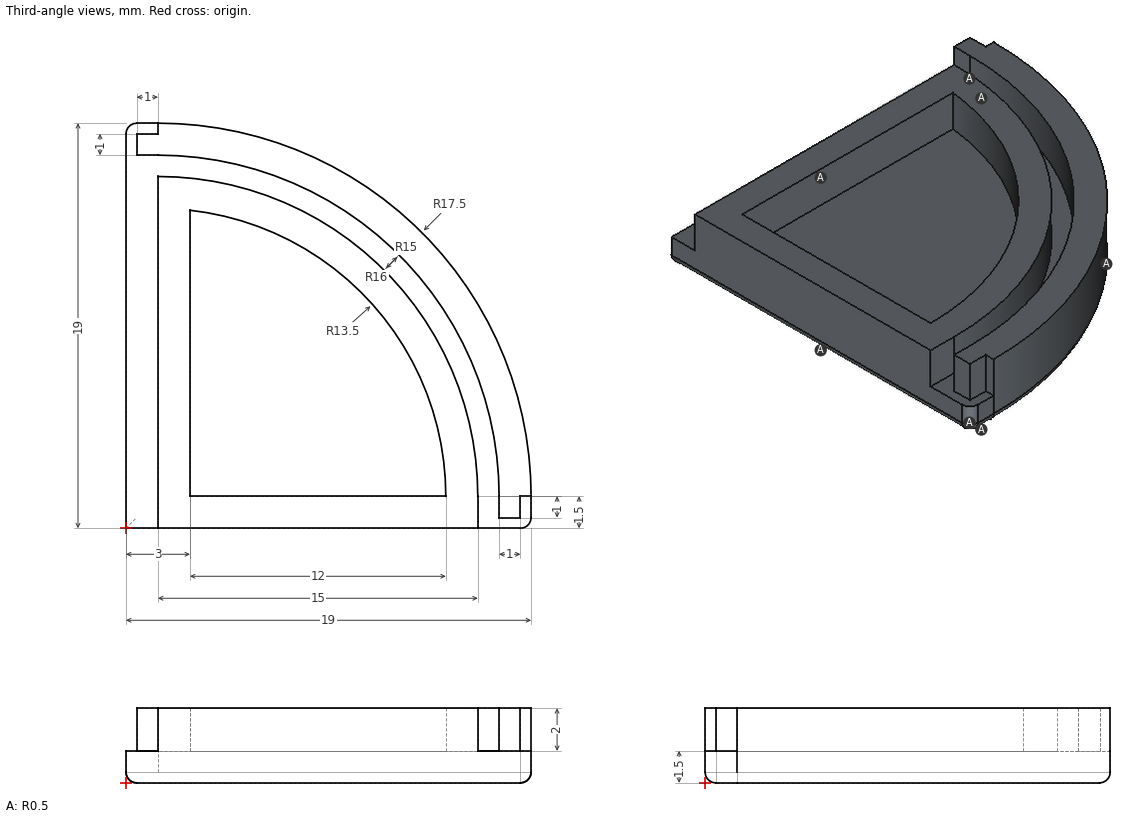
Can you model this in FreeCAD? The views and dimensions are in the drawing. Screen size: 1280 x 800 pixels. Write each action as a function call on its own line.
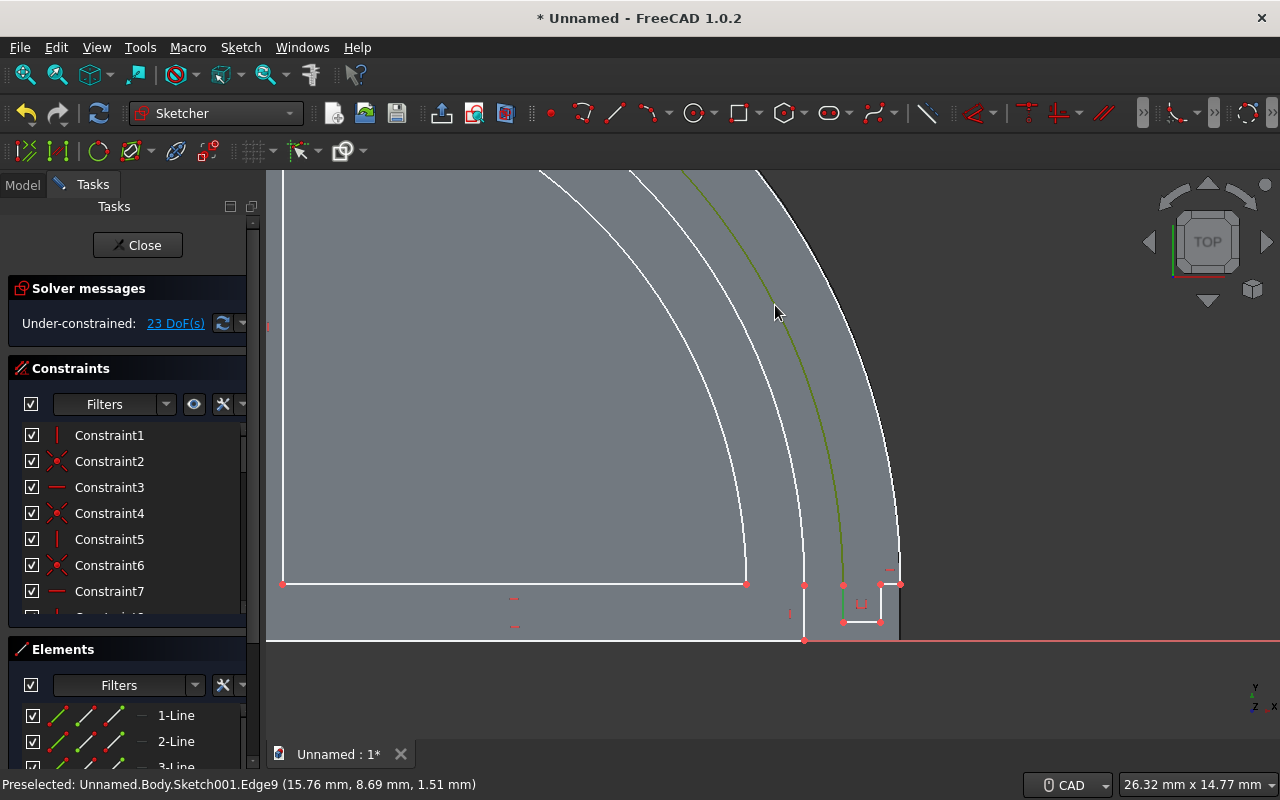
key(t)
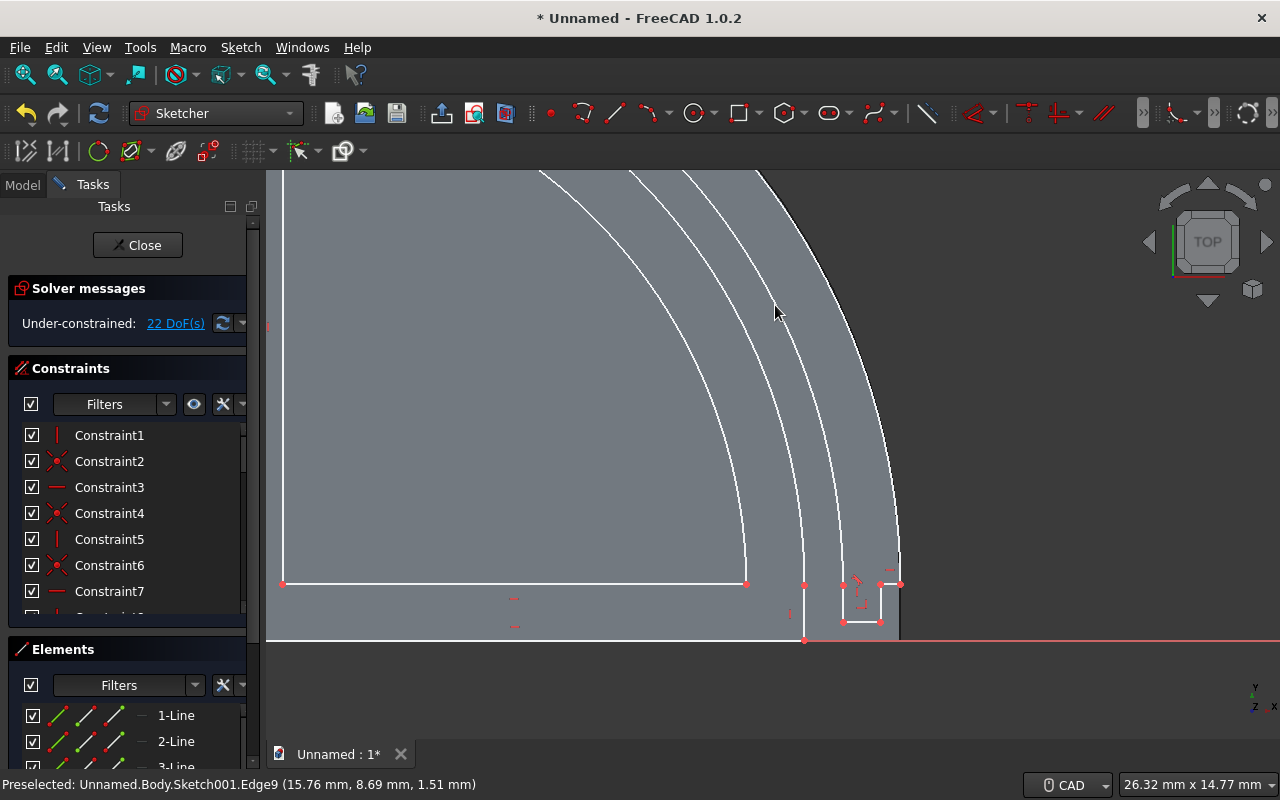
click(804, 624)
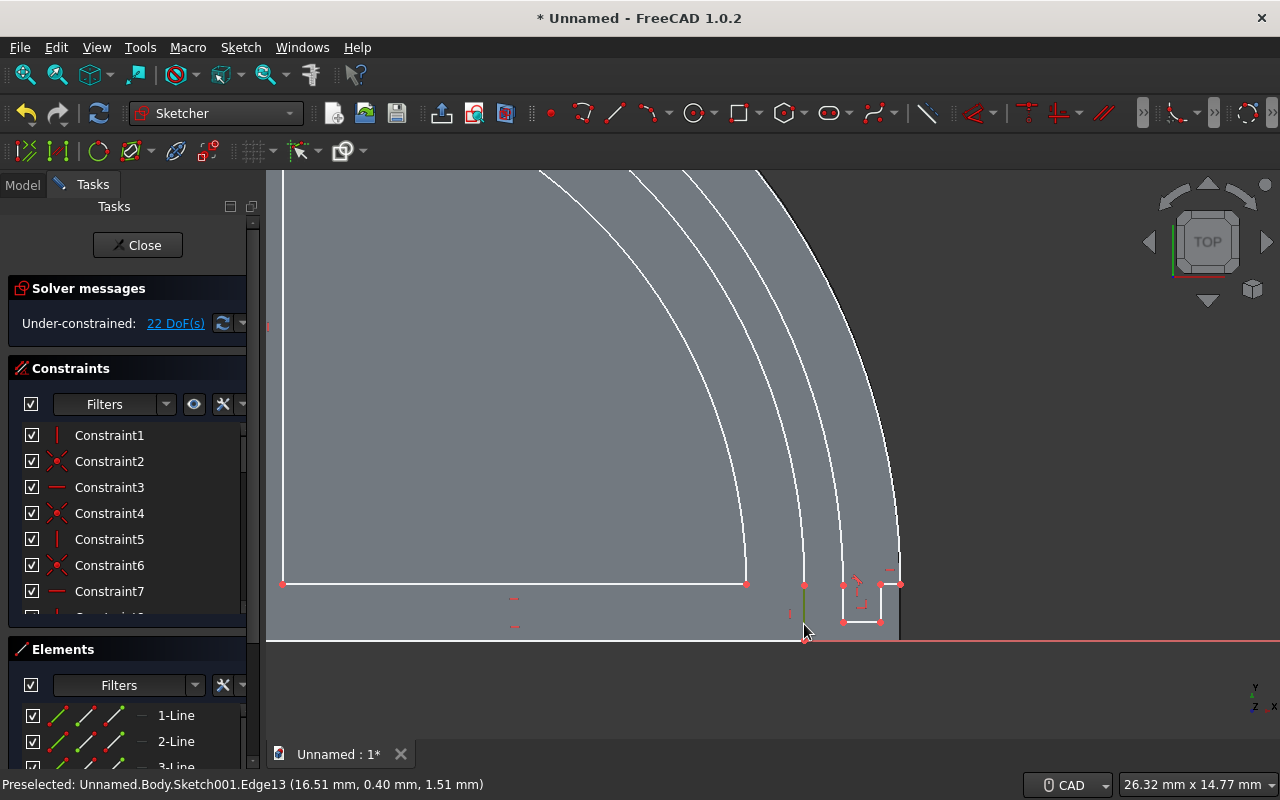
click(742, 323)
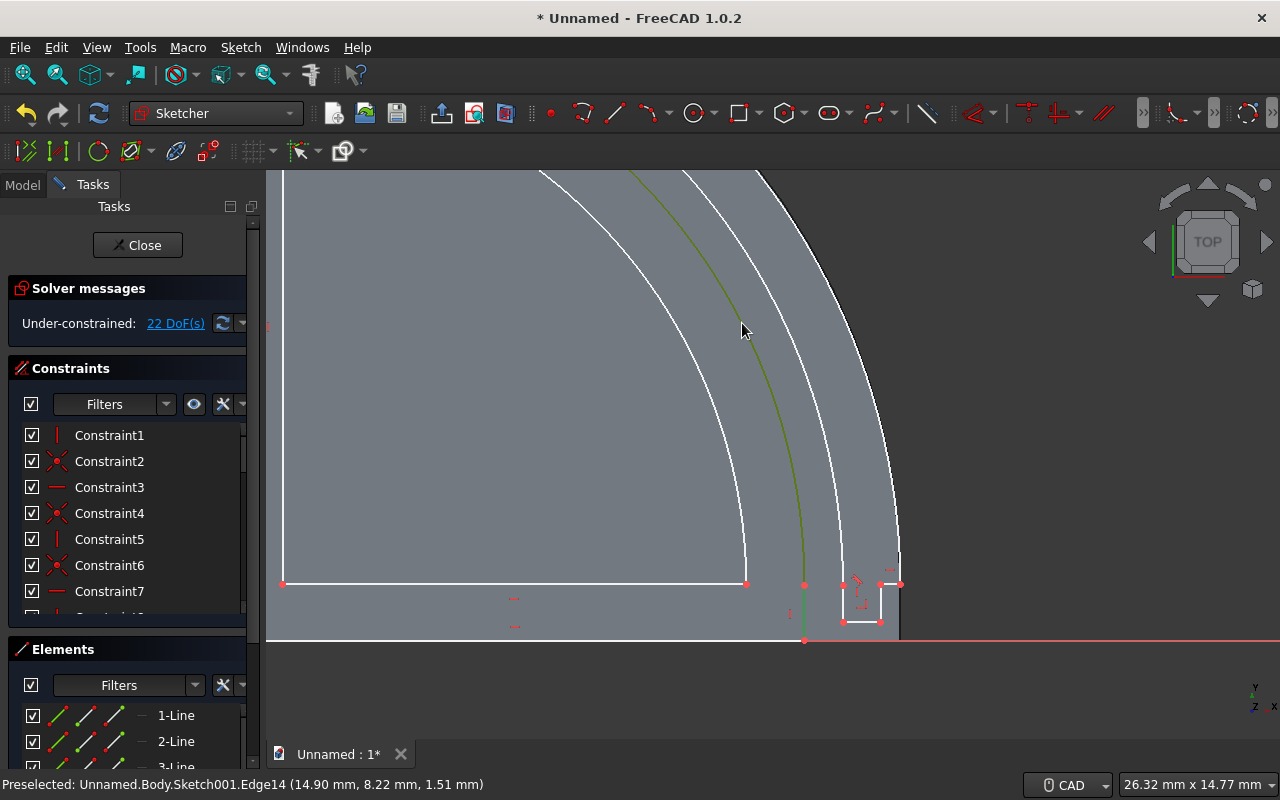
key(t)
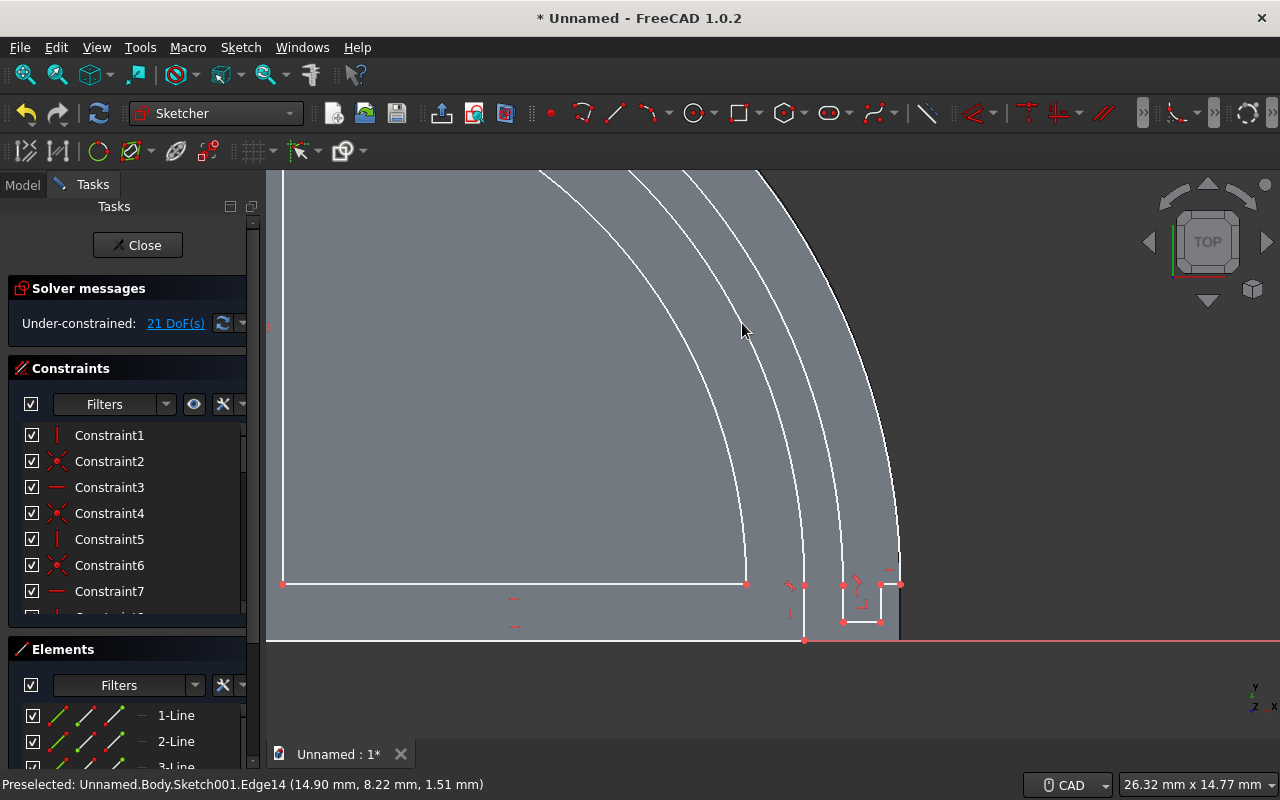
click(775, 304)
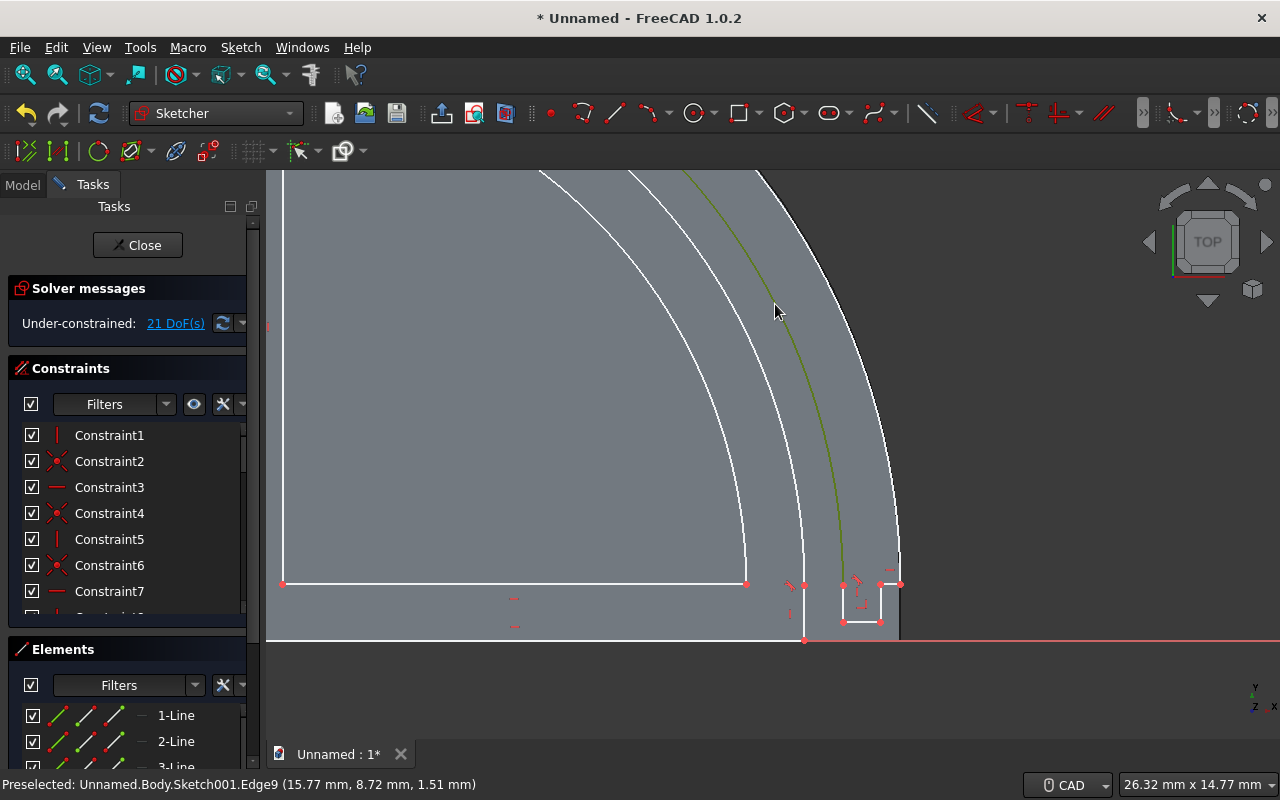
click(826, 279)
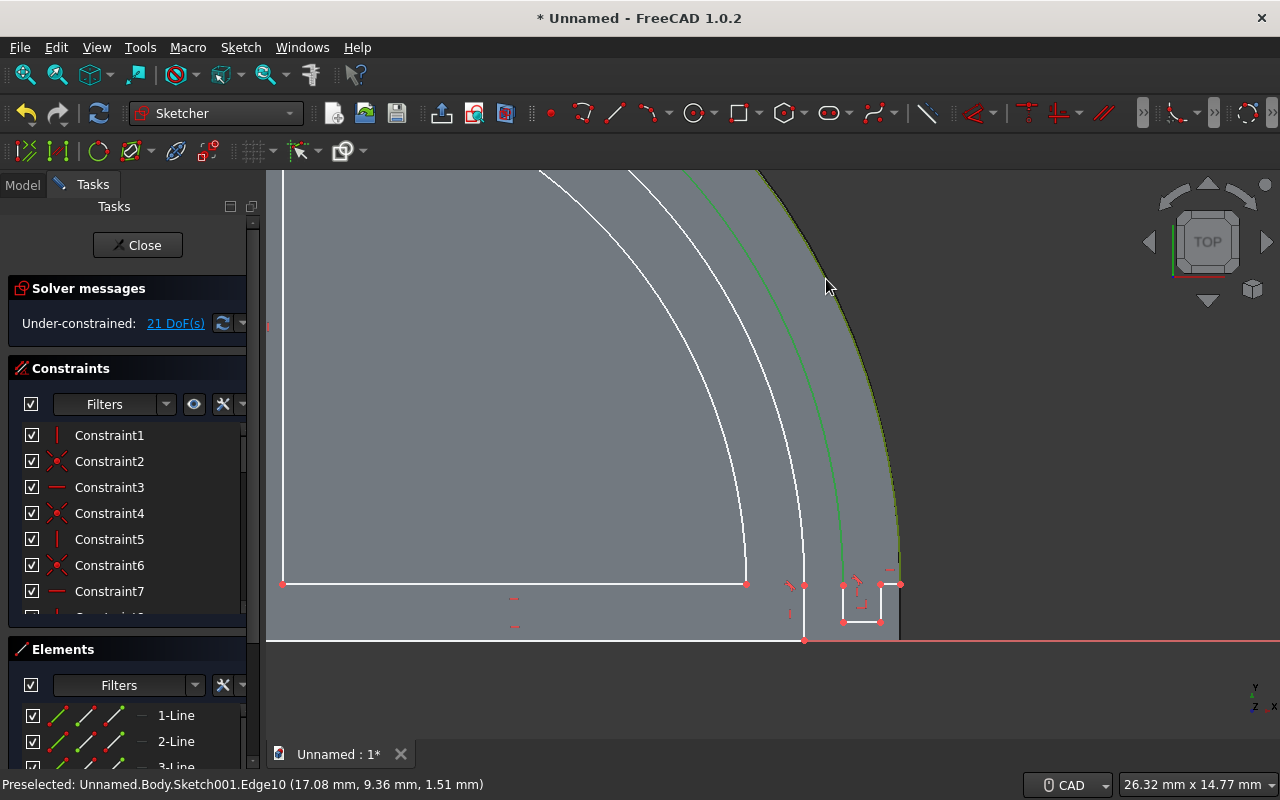
key(c)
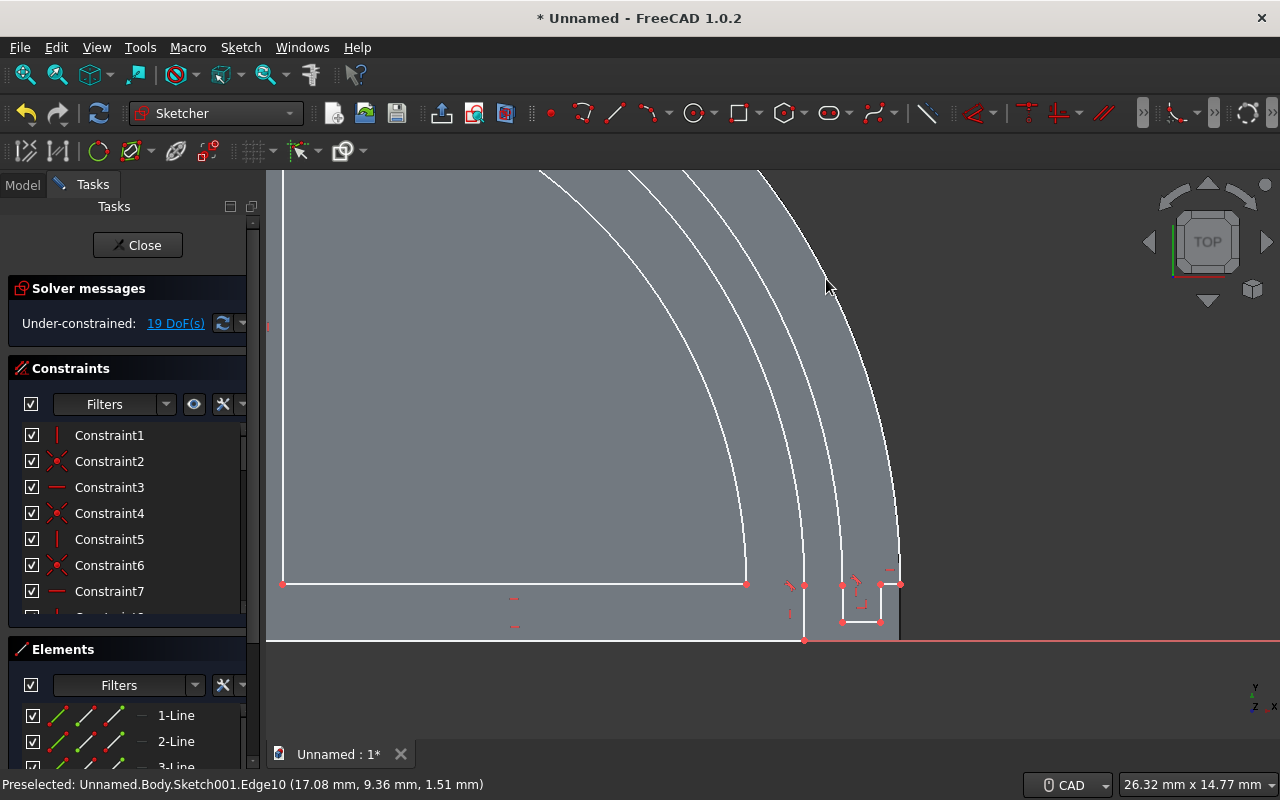
click(775, 304)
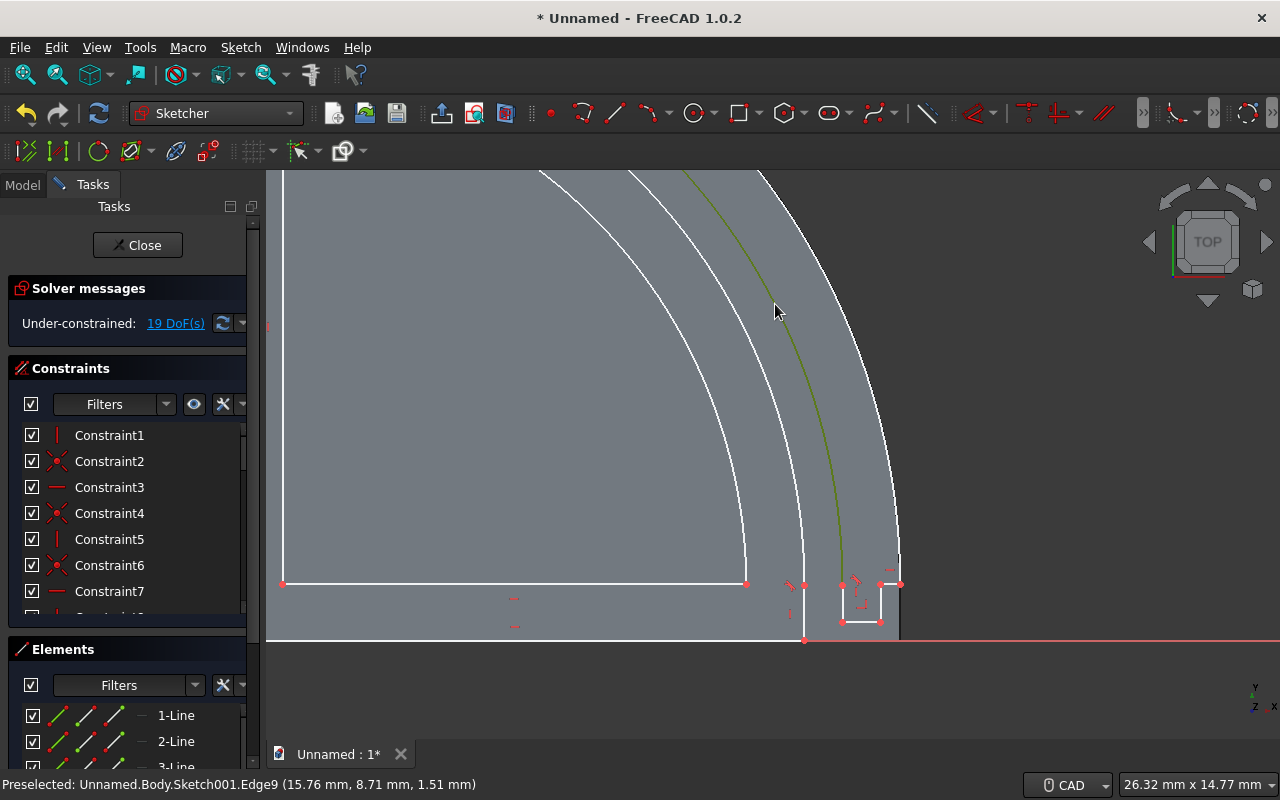
click(741, 323)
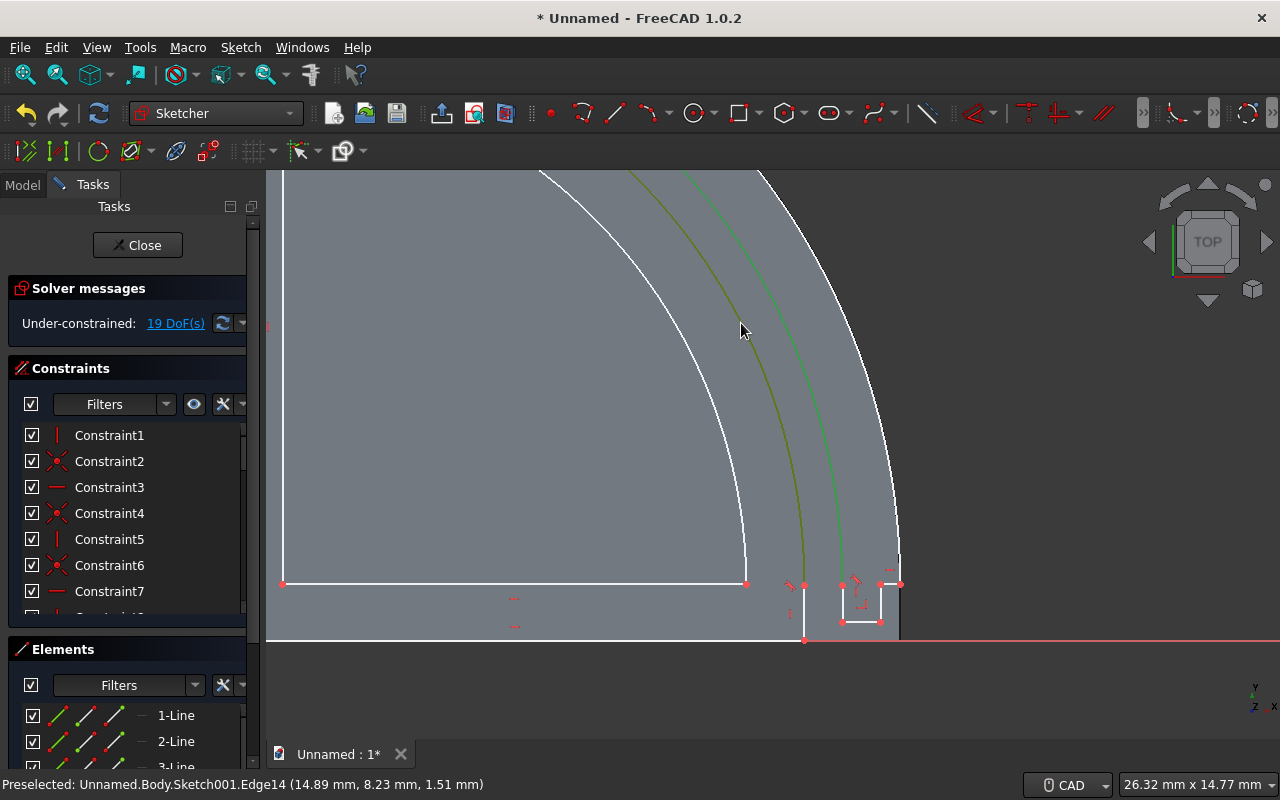
key(c)